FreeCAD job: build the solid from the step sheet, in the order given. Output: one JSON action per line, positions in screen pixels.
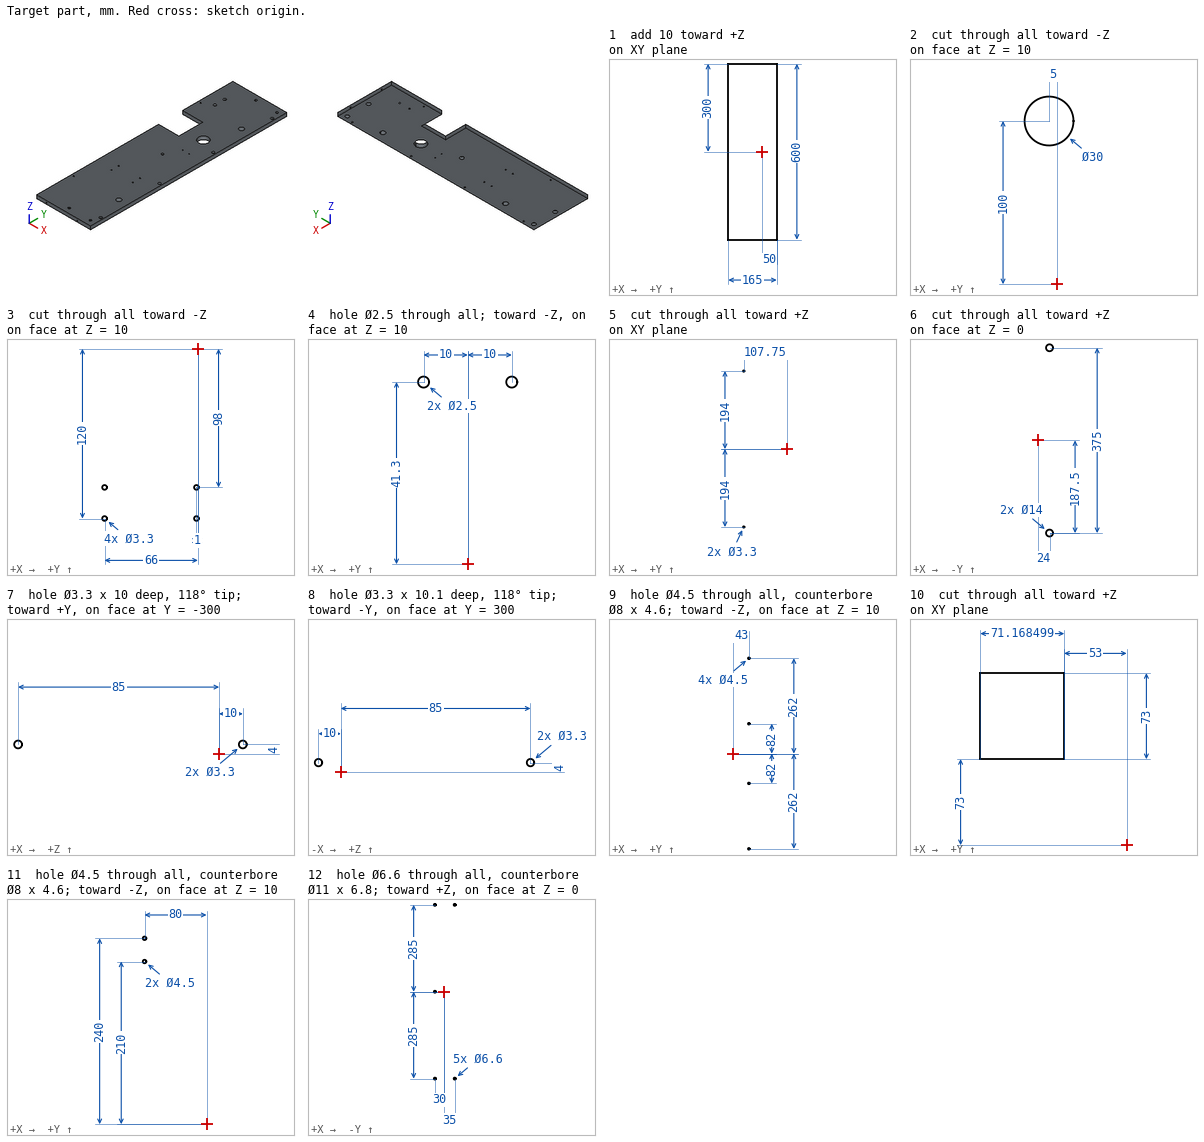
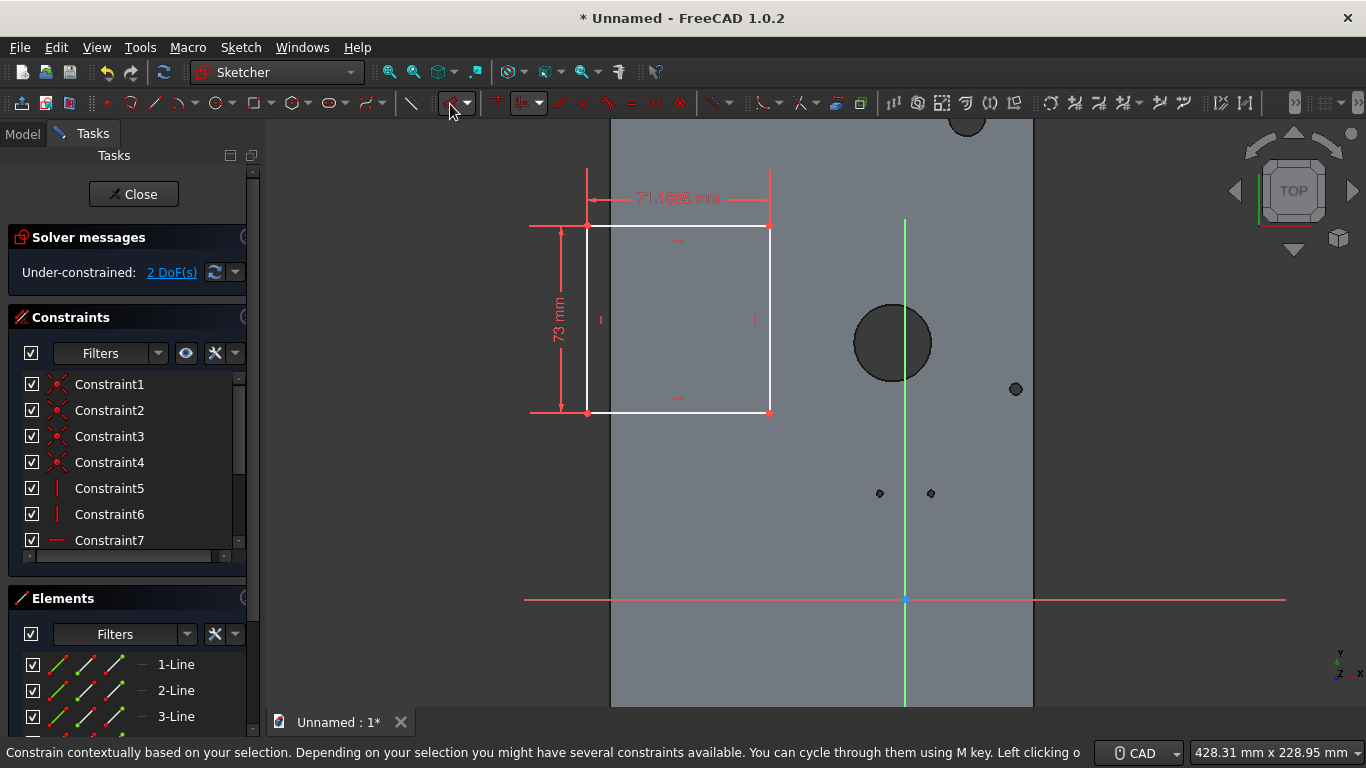
{"action": "left_click", "coordinate": [587, 413]}
{"action": "left_click", "coordinate": [939, 507]}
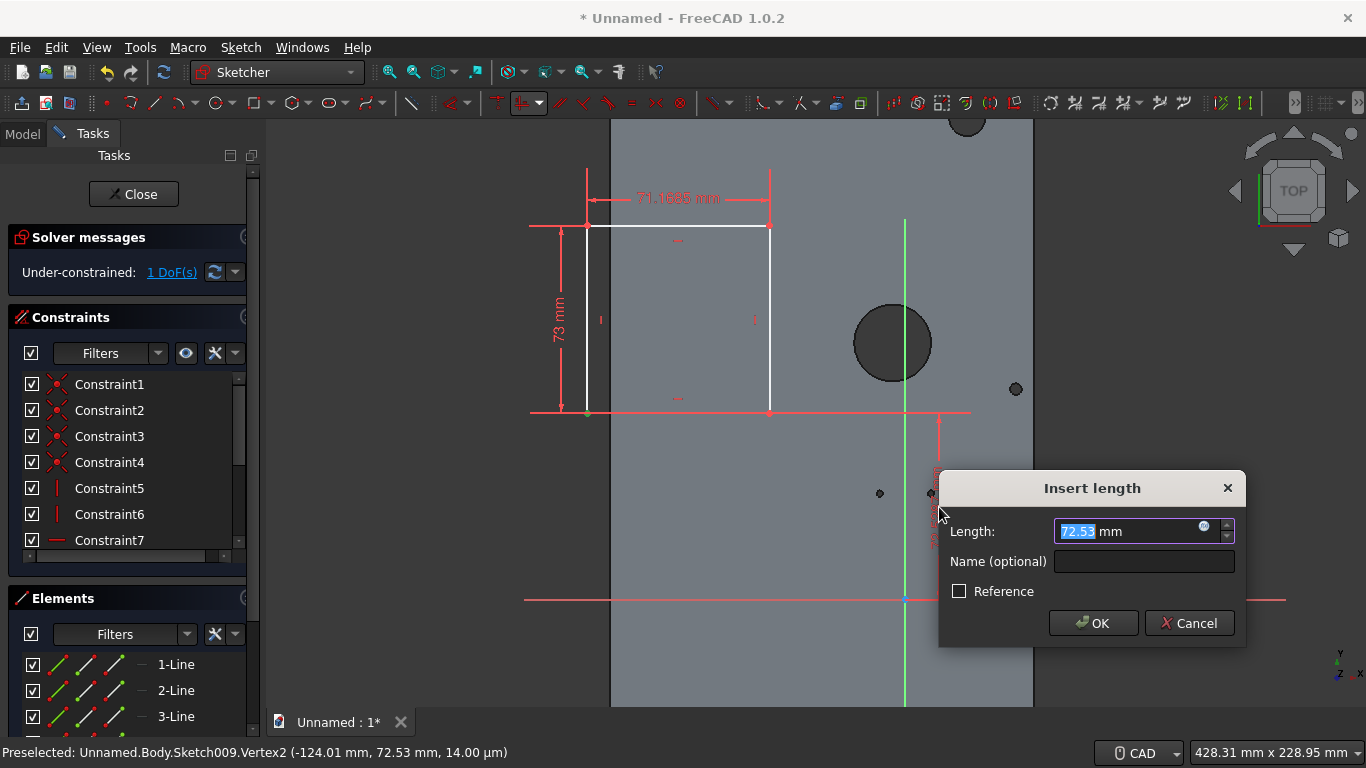
{"action": "type", "text": "73"}
{"action": "key", "text": "Return"}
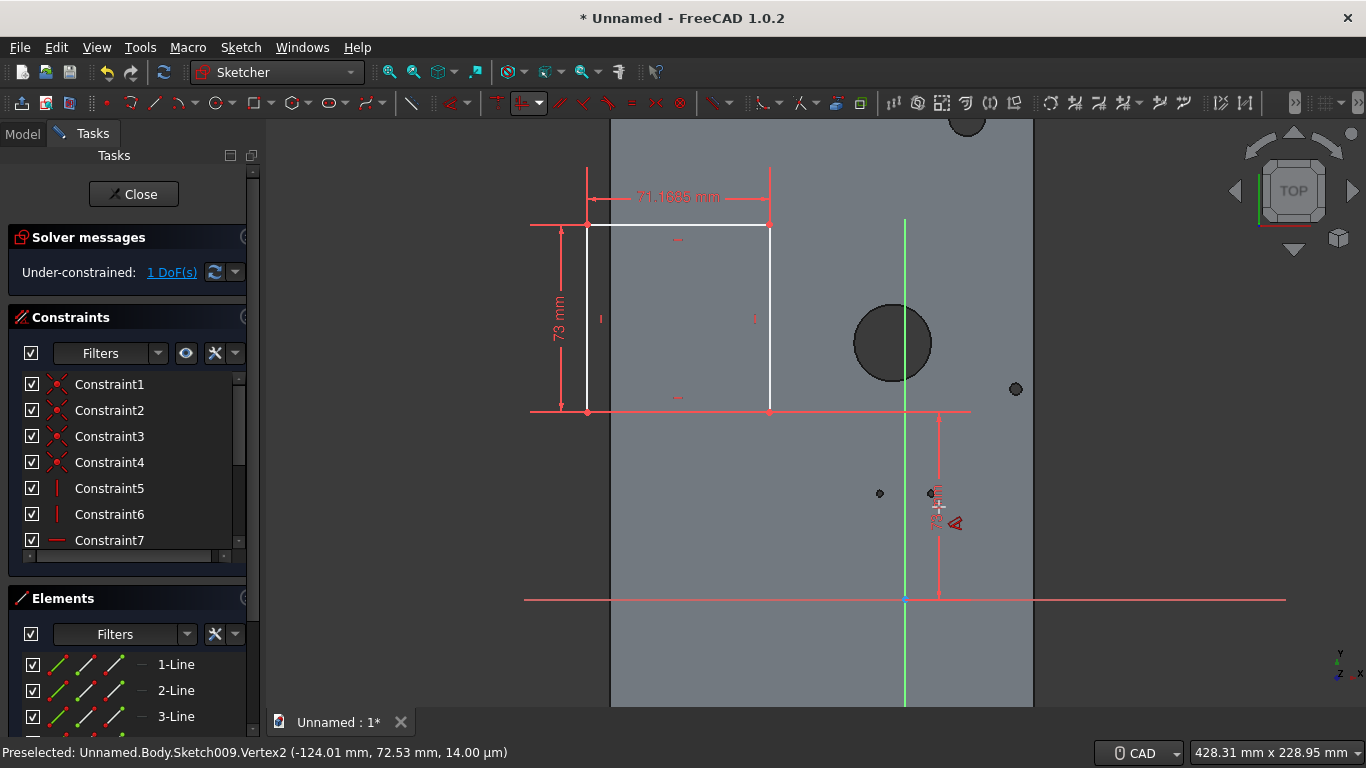
{"action": "left_click", "coordinate": [770, 412]}
{"action": "left_click", "coordinate": [838, 634]}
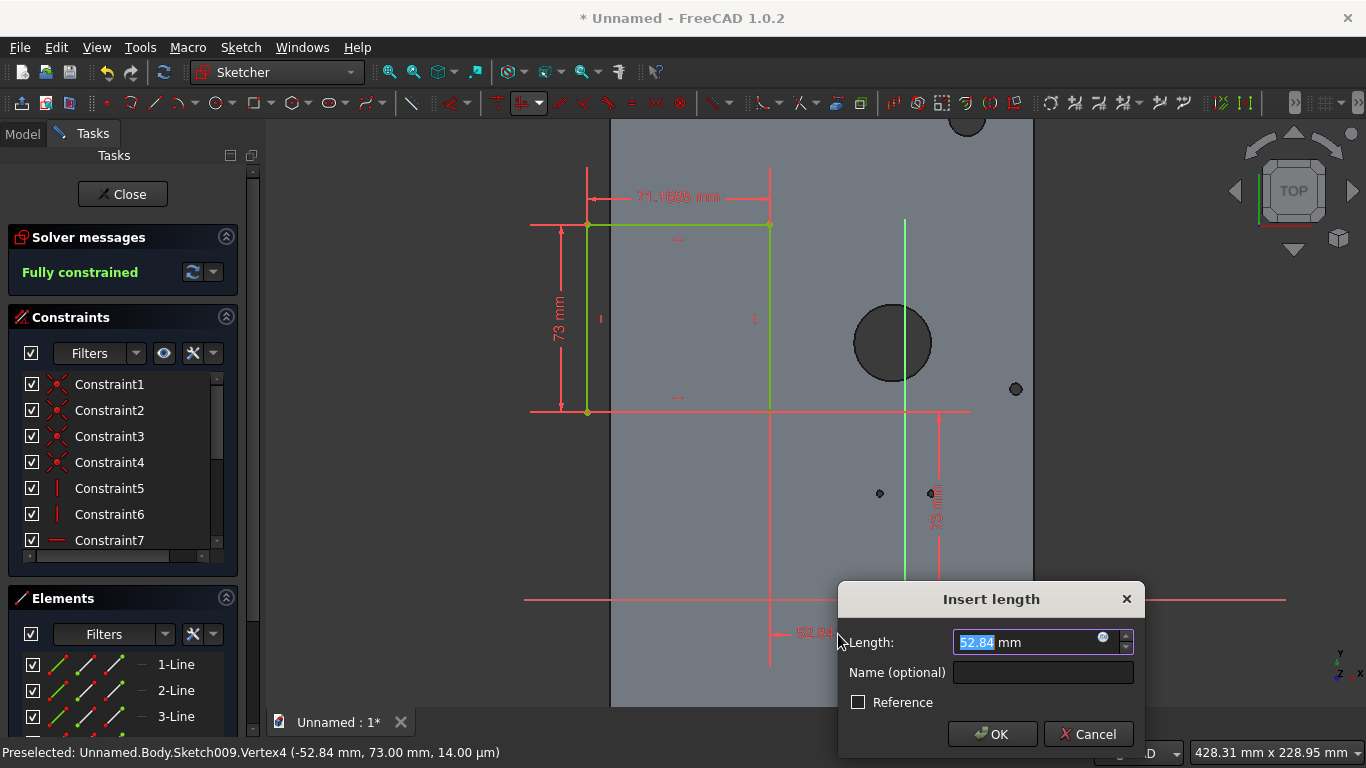
{"action": "type", "text": "53"}
{"action": "key", "text": "Return"}
{"action": "key", "text": "Escape"}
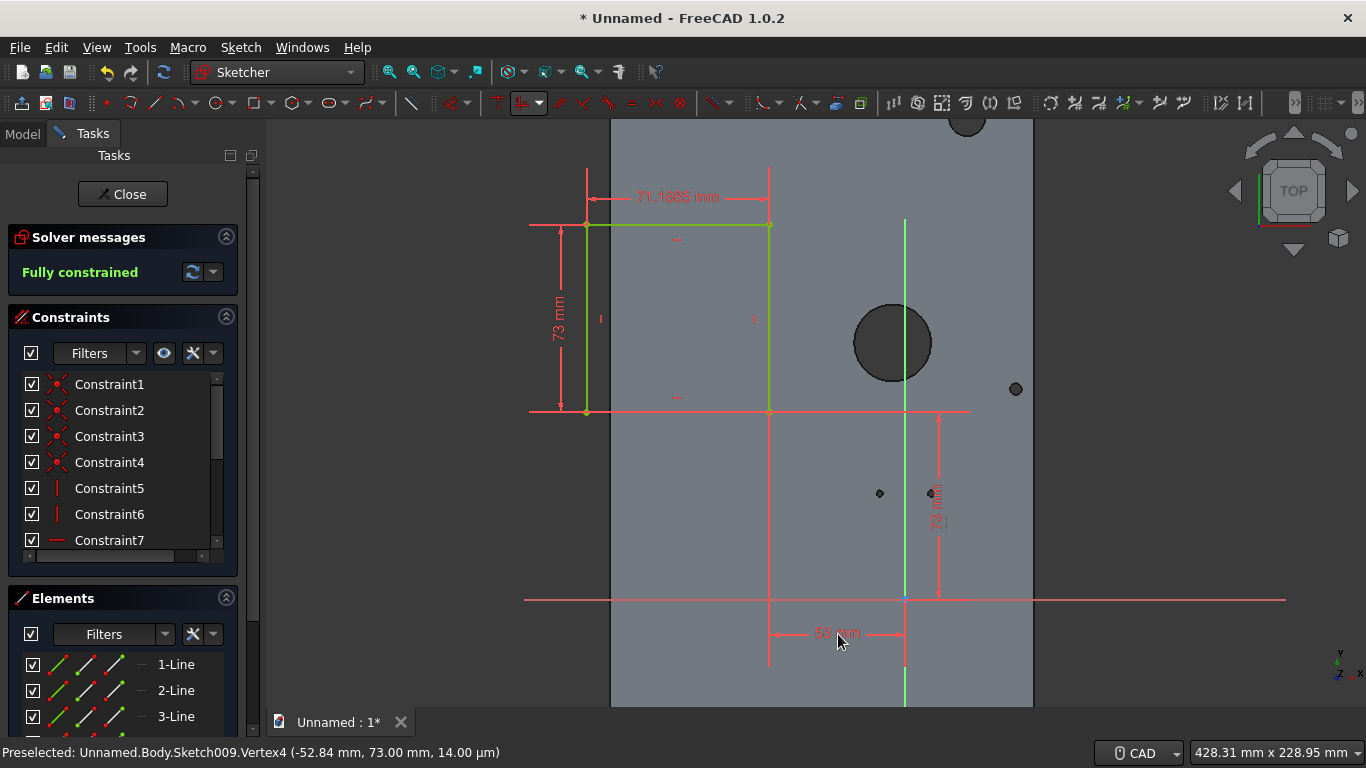
{"action": "left_click", "coordinate": [123, 194]}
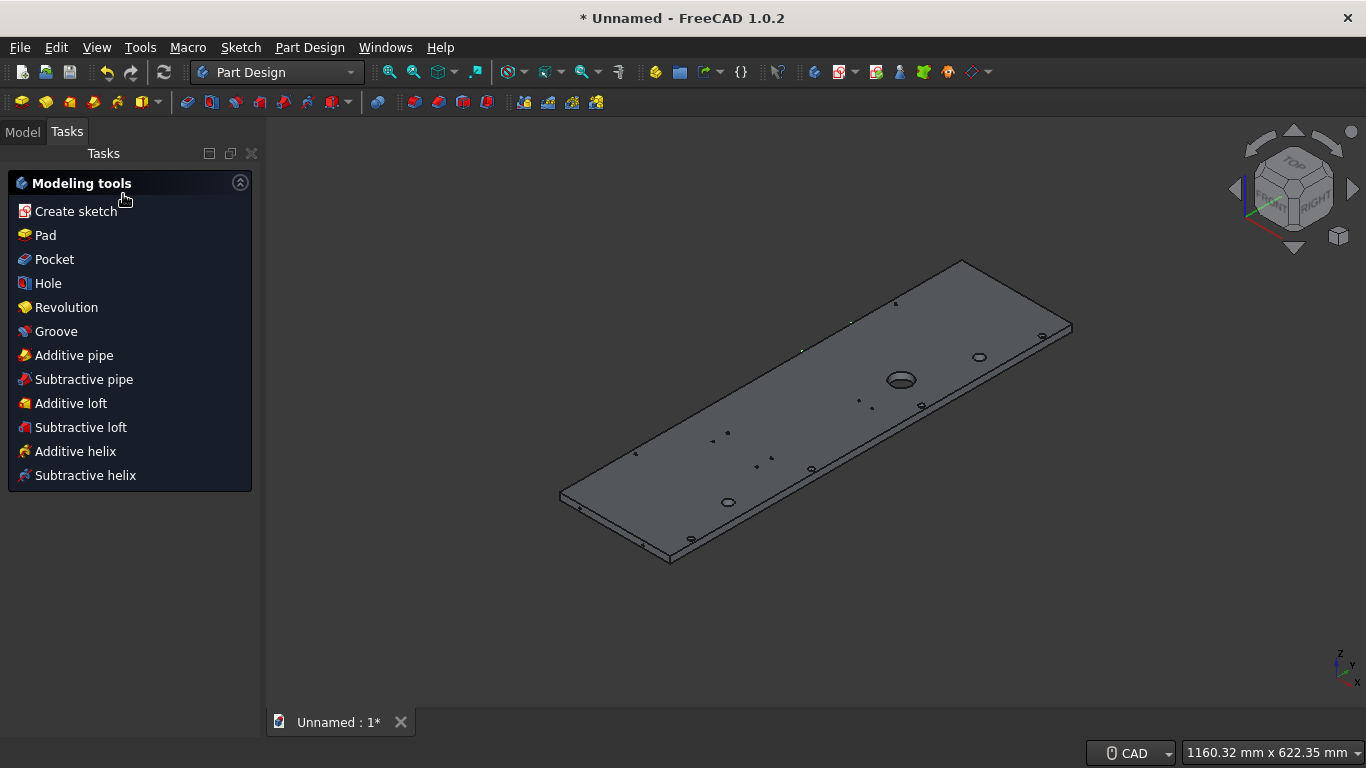
{"action": "left_click", "coordinate": [188, 102]}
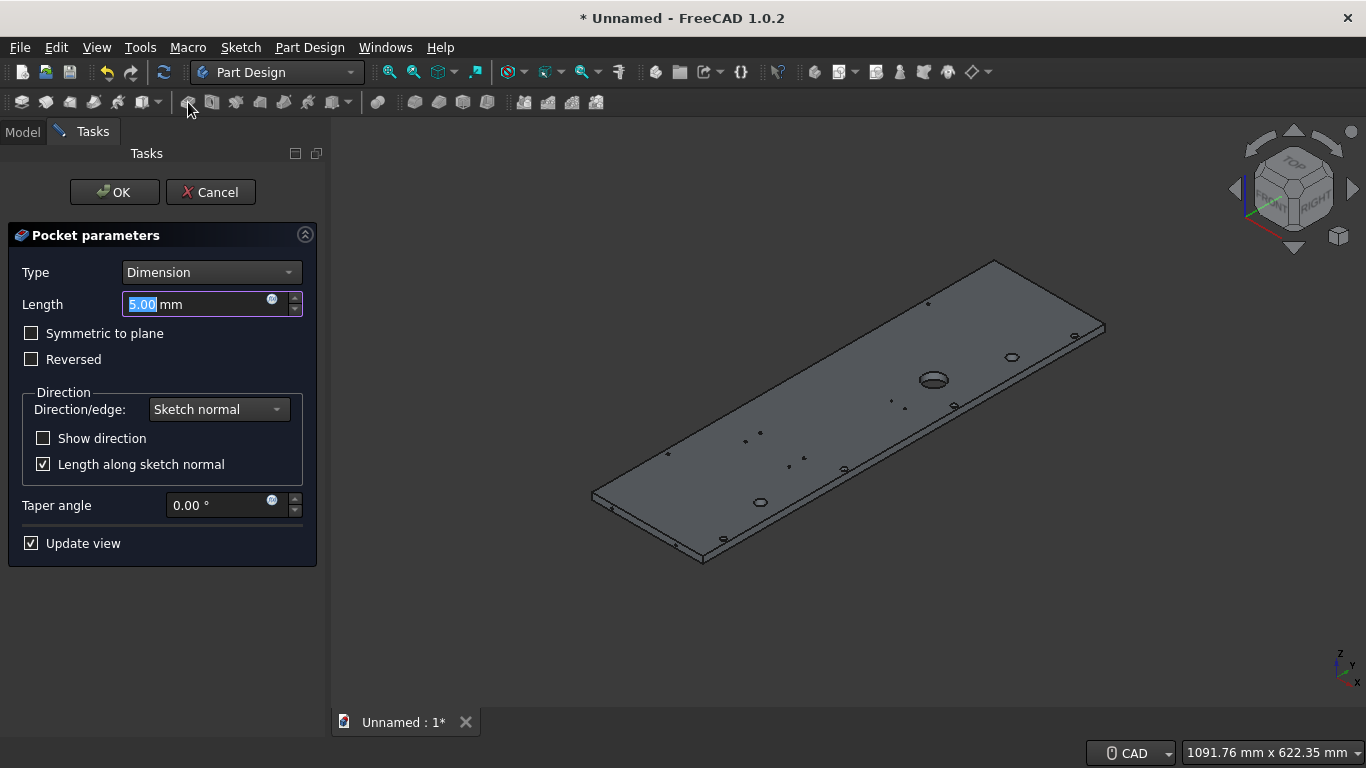
{"action": "left_click", "coordinate": [212, 272]}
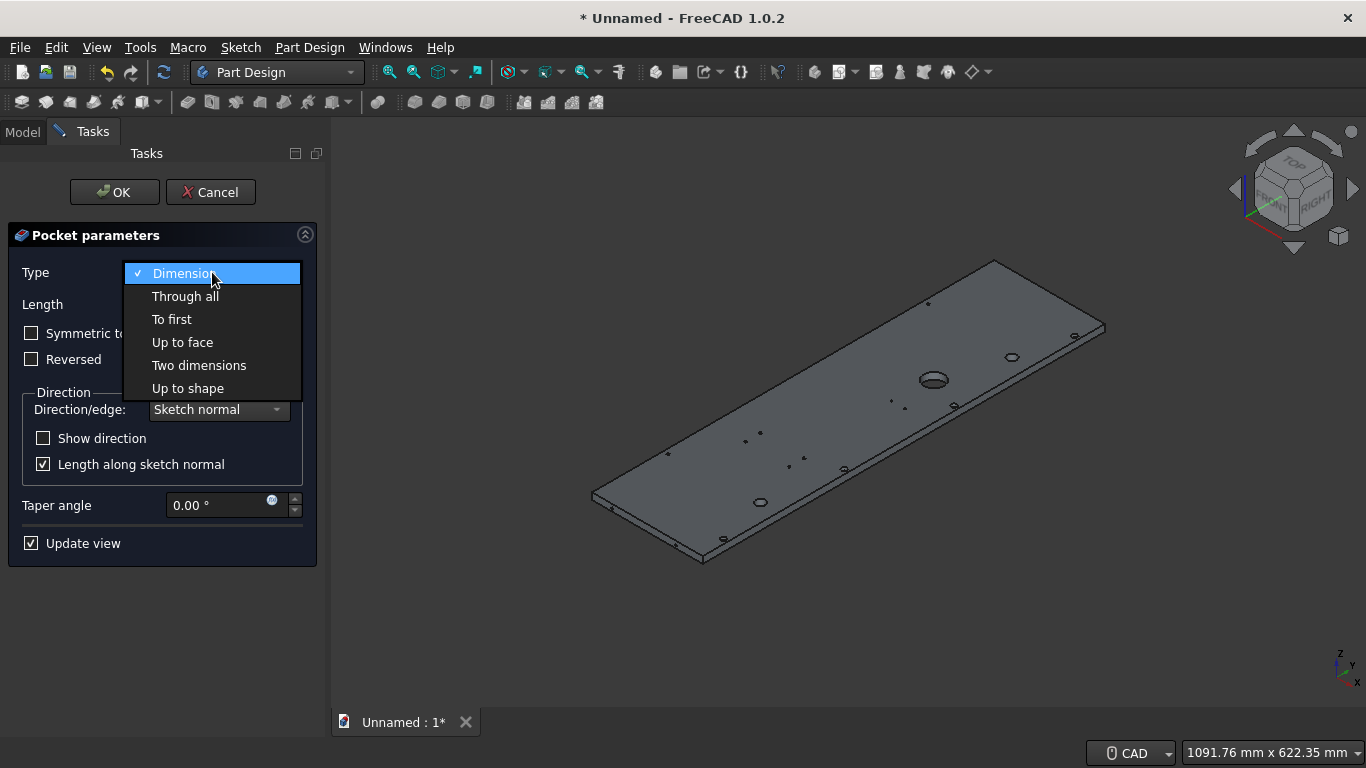
{"action": "left_click", "coordinate": [212, 296]}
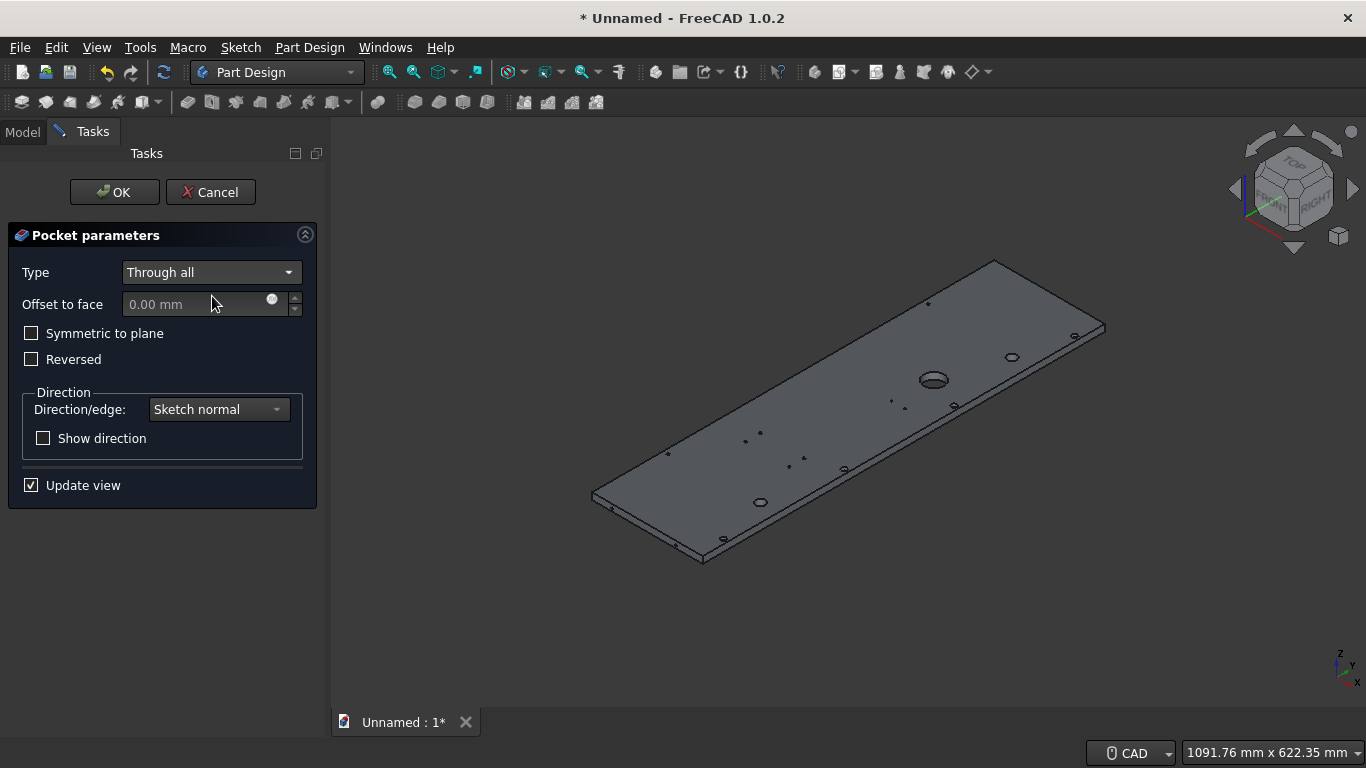
{"action": "left_click", "coordinate": [30, 359]}